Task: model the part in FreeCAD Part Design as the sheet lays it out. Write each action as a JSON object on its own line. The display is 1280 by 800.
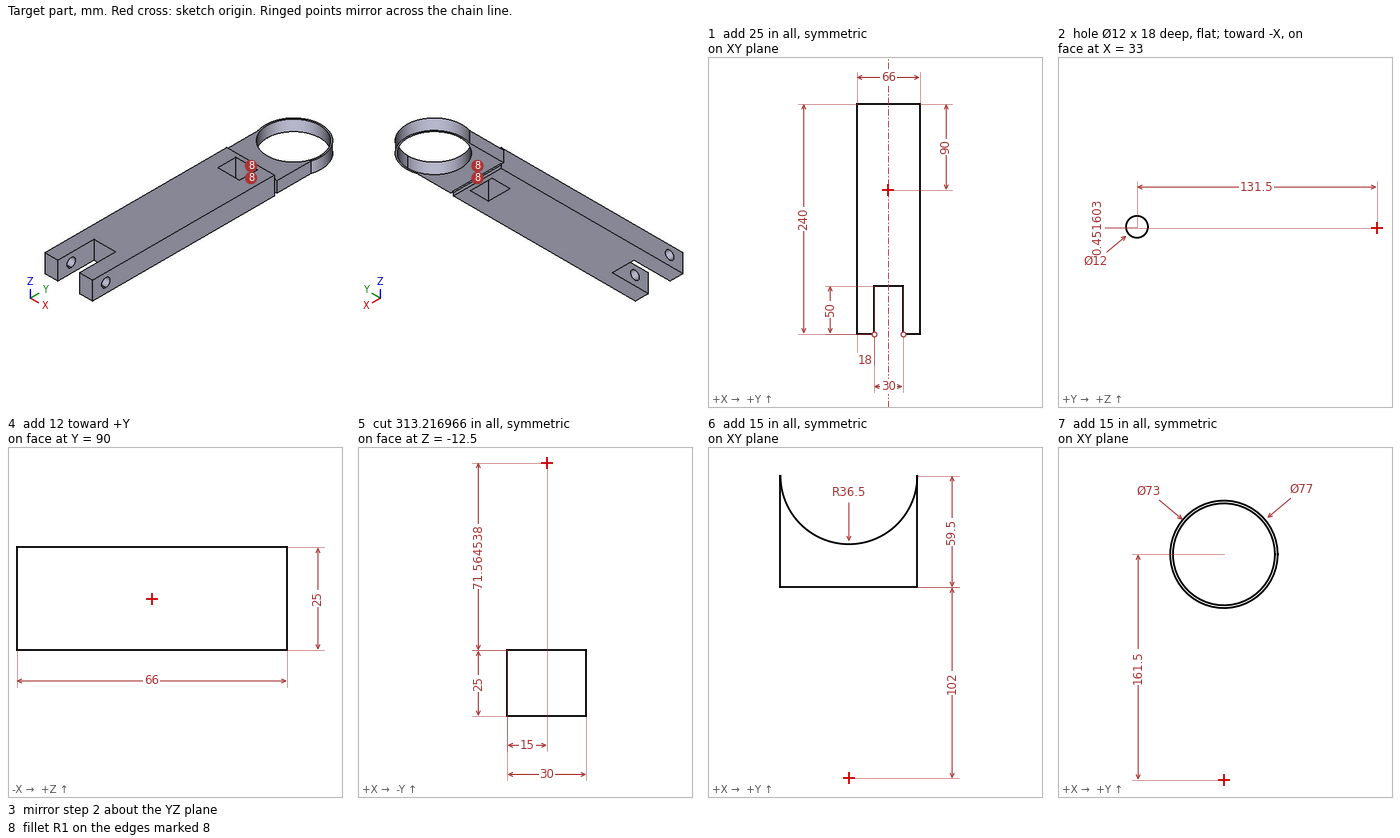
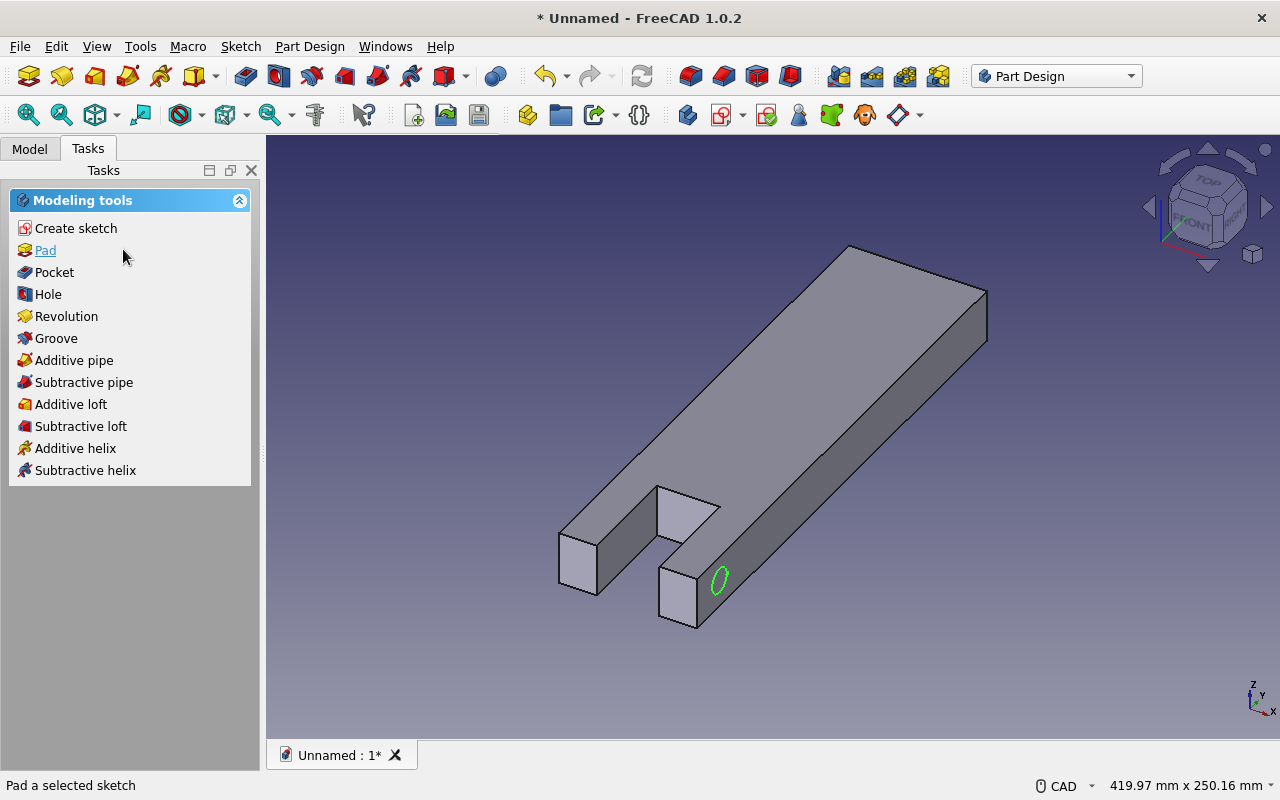
{"action": "left_click", "coordinate": [279, 76]}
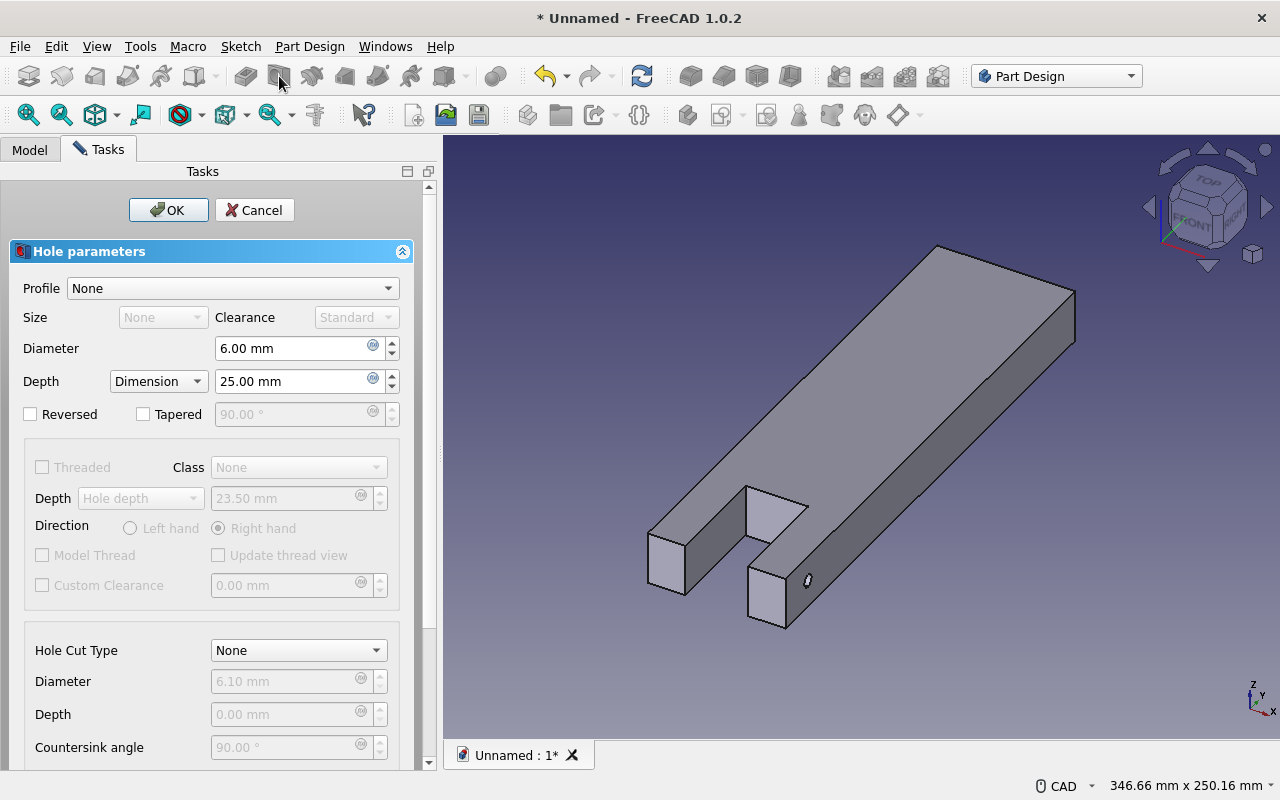
{"action": "triple_click", "coordinate": [300, 348]}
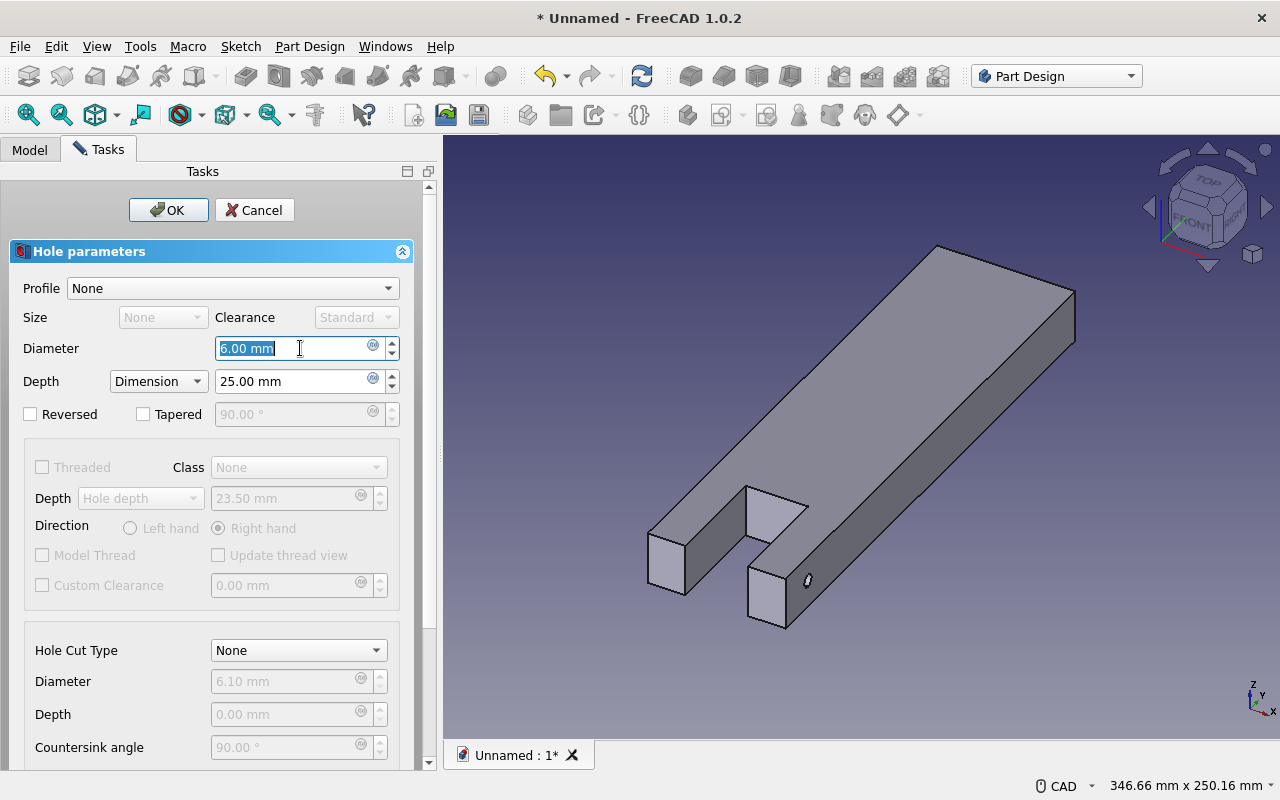
{"action": "type", "text": "12"}
{"action": "key", "text": "Tab"}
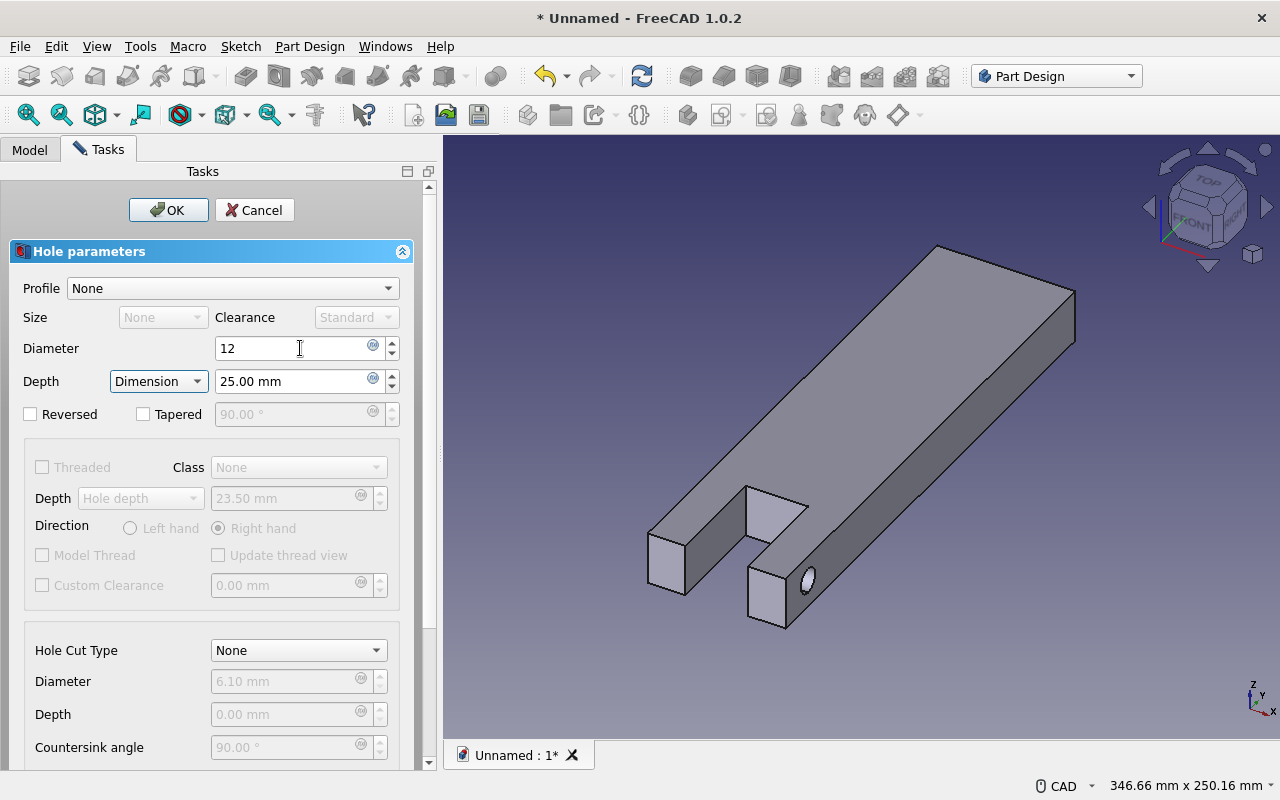
{"action": "triple_click", "coordinate": [300, 382]}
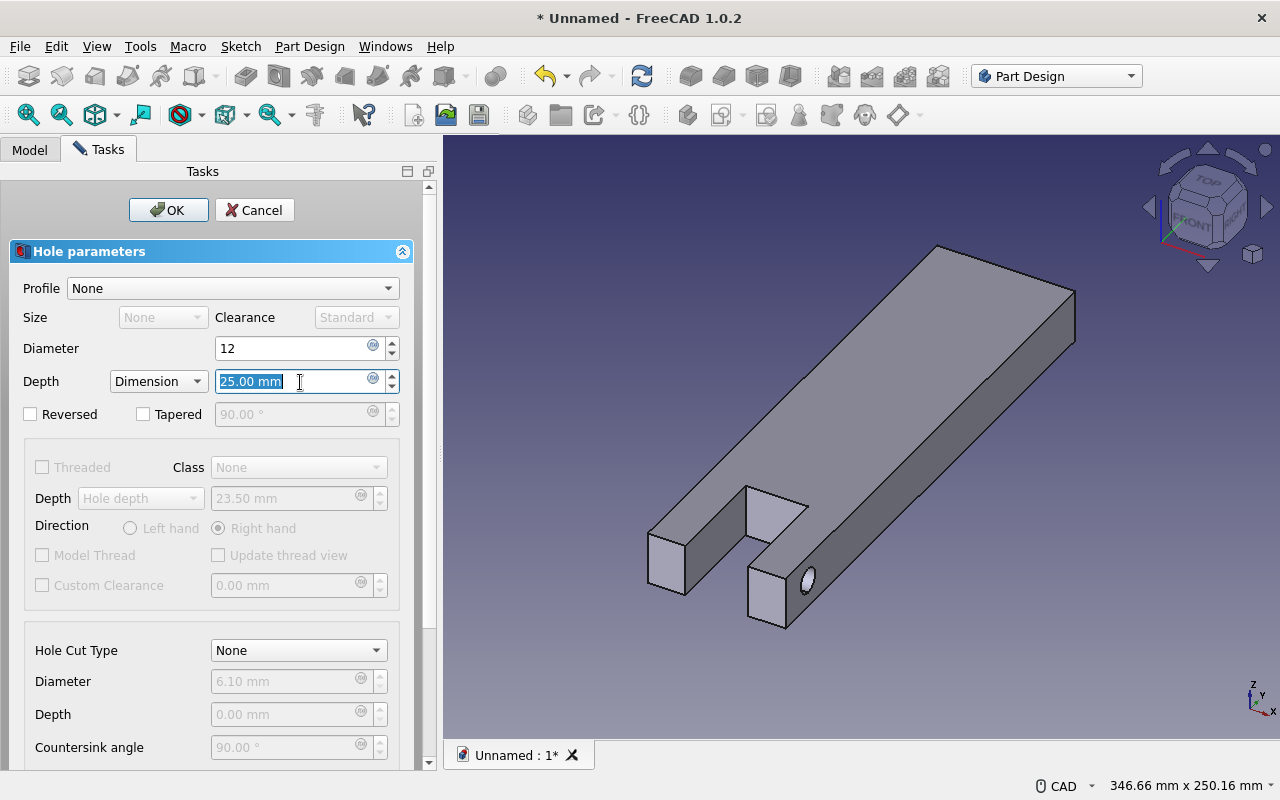
{"action": "type", "text": "18"}
{"action": "key", "text": "Tab"}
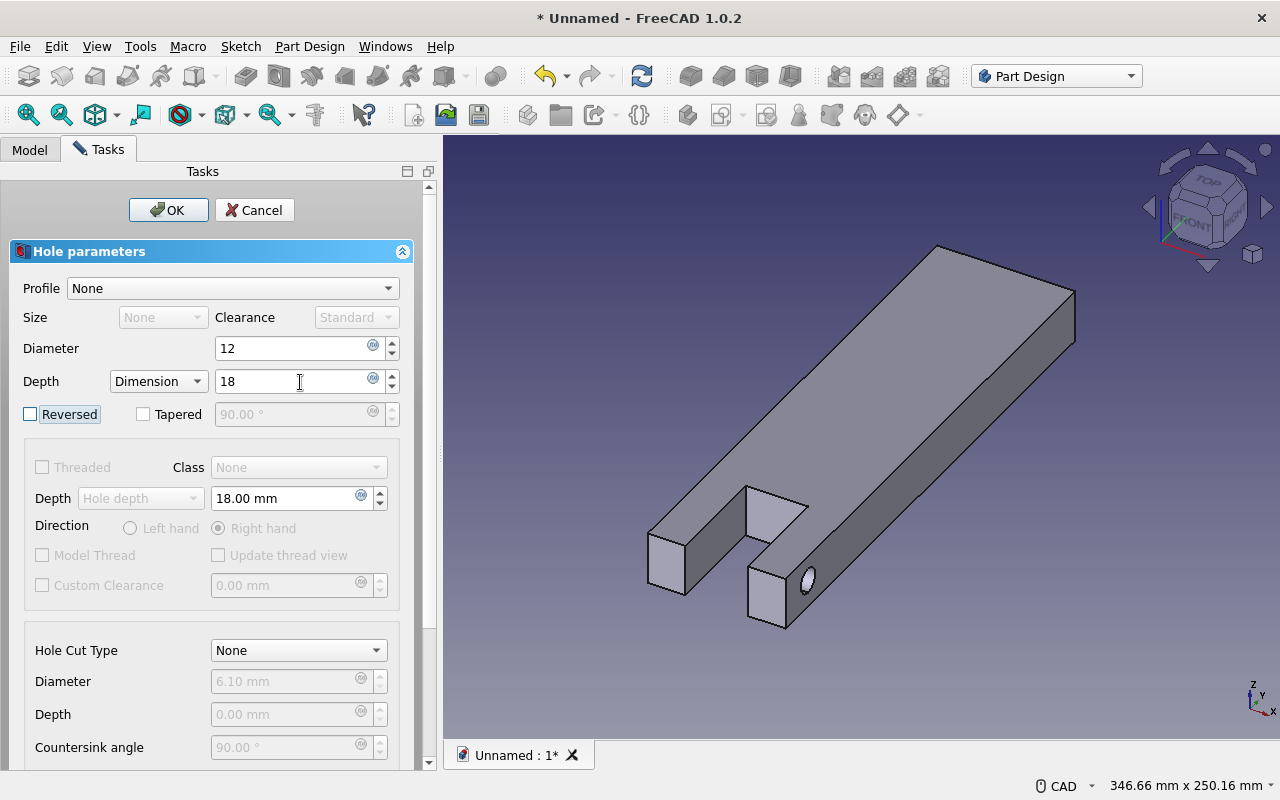
{"action": "scroll", "coordinate": [429, 476], "scroll_direction": "down", "scroll_amount": 3}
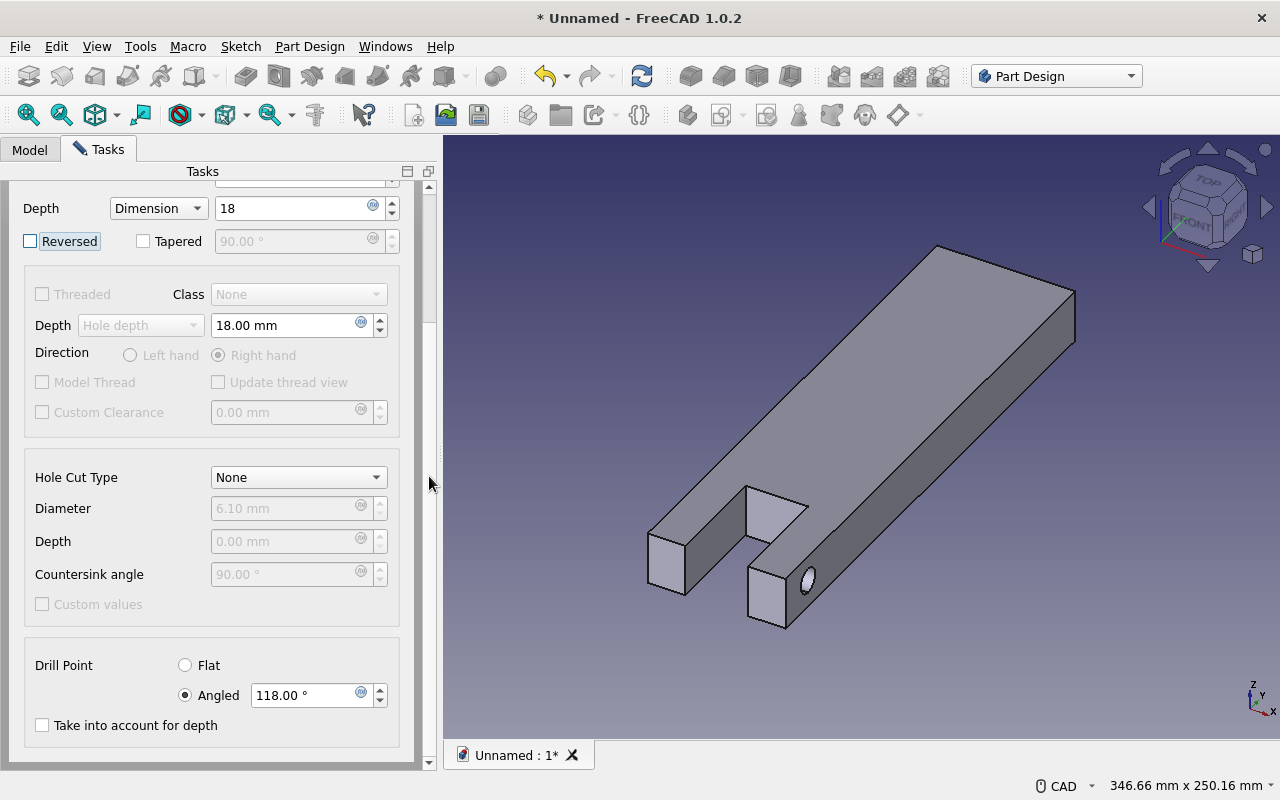
{"action": "left_click", "coordinate": [186, 663]}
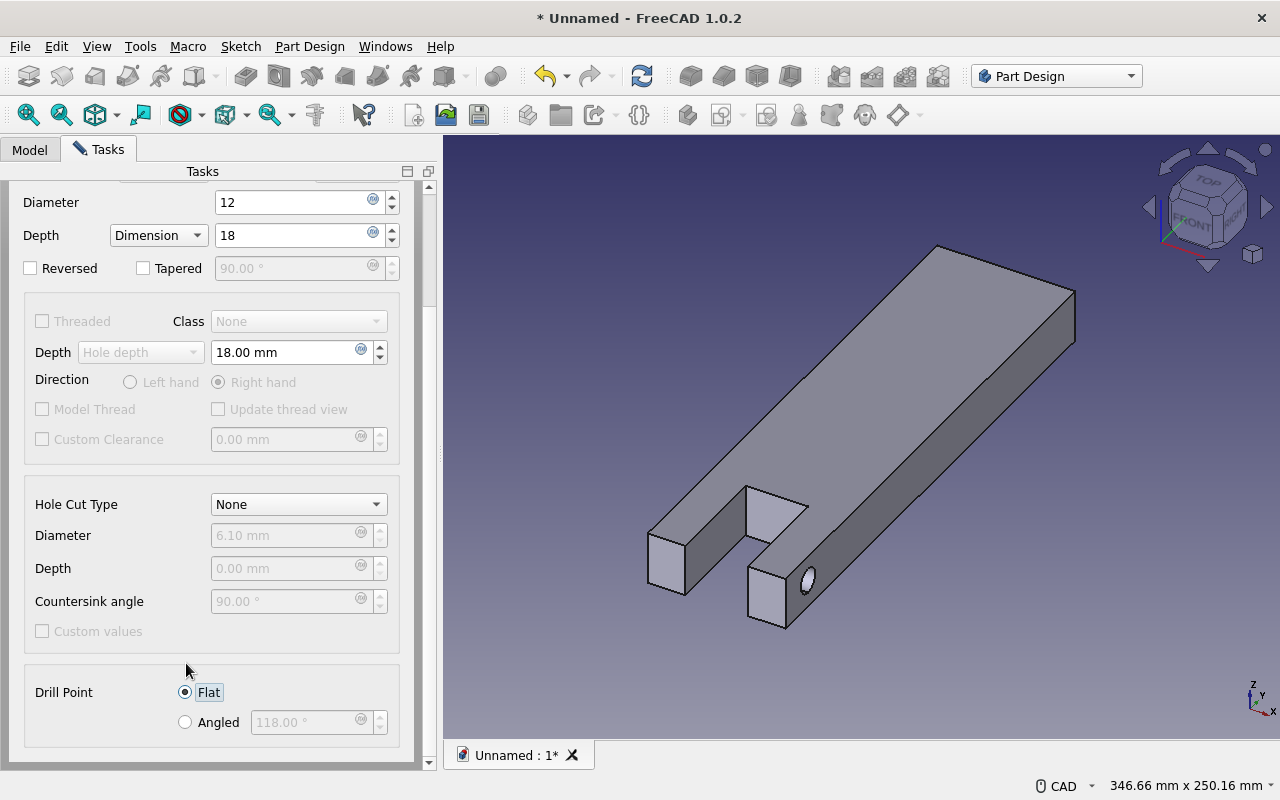
{"action": "scroll", "coordinate": [429, 476], "scroll_direction": "up", "scroll_amount": 4}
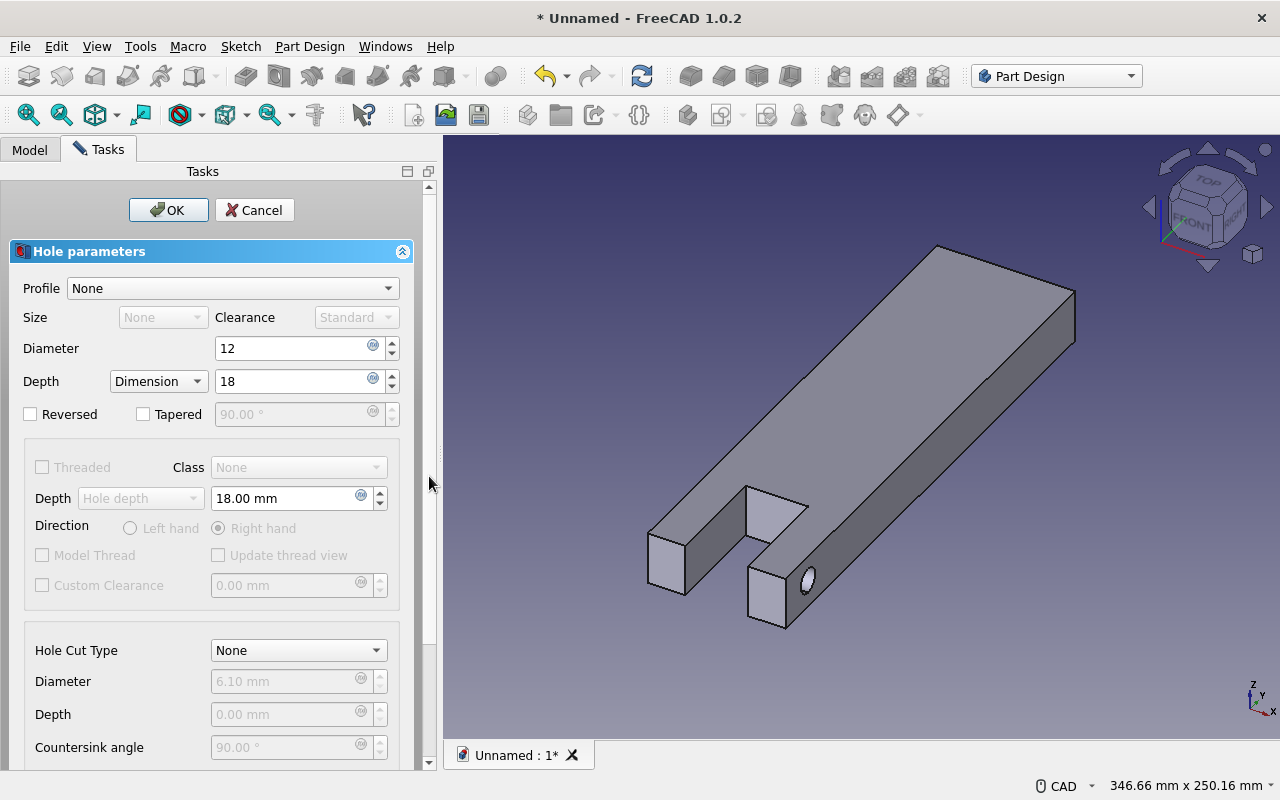
{"action": "left_click", "coordinate": [169, 210]}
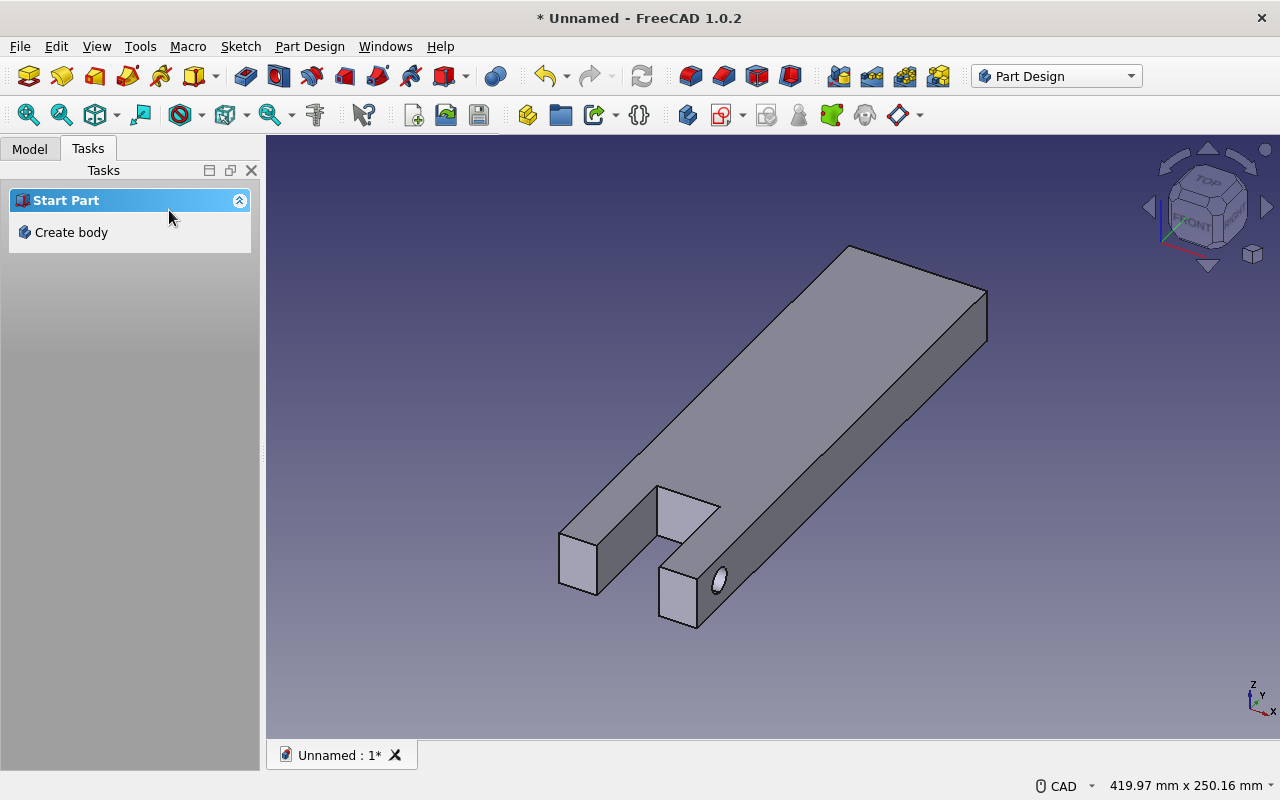
{"action": "left_click", "coordinate": [30, 148]}